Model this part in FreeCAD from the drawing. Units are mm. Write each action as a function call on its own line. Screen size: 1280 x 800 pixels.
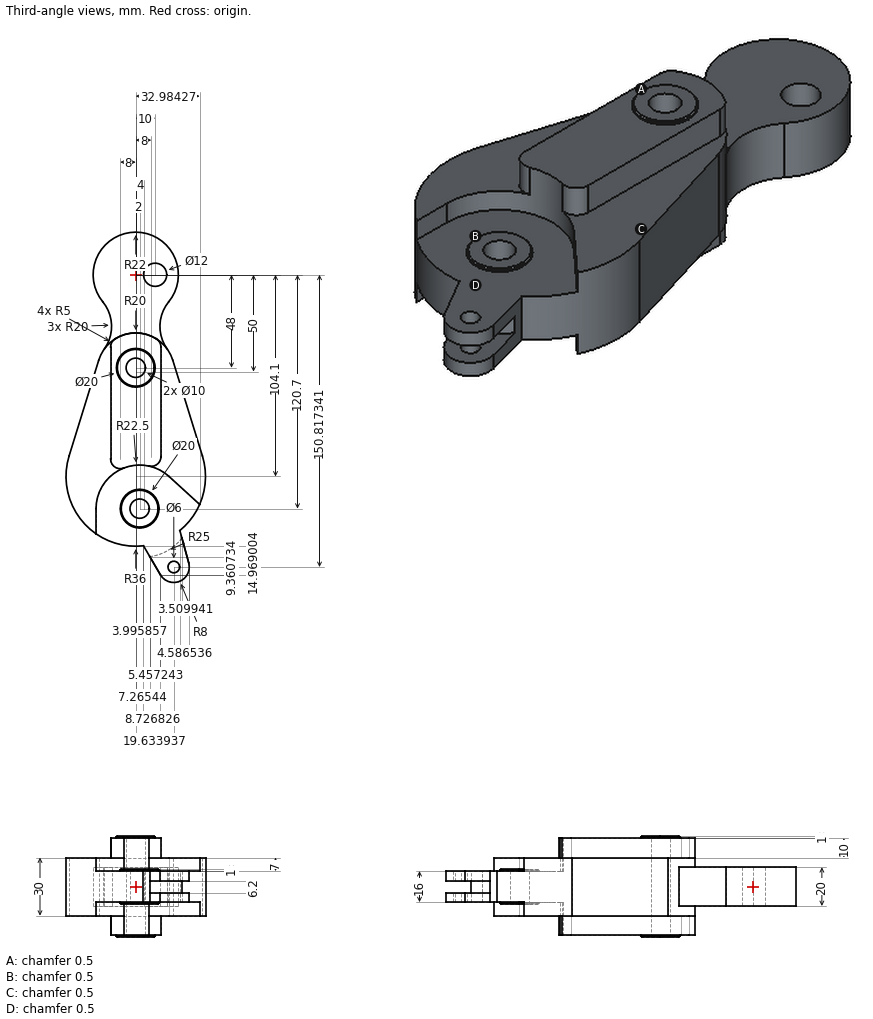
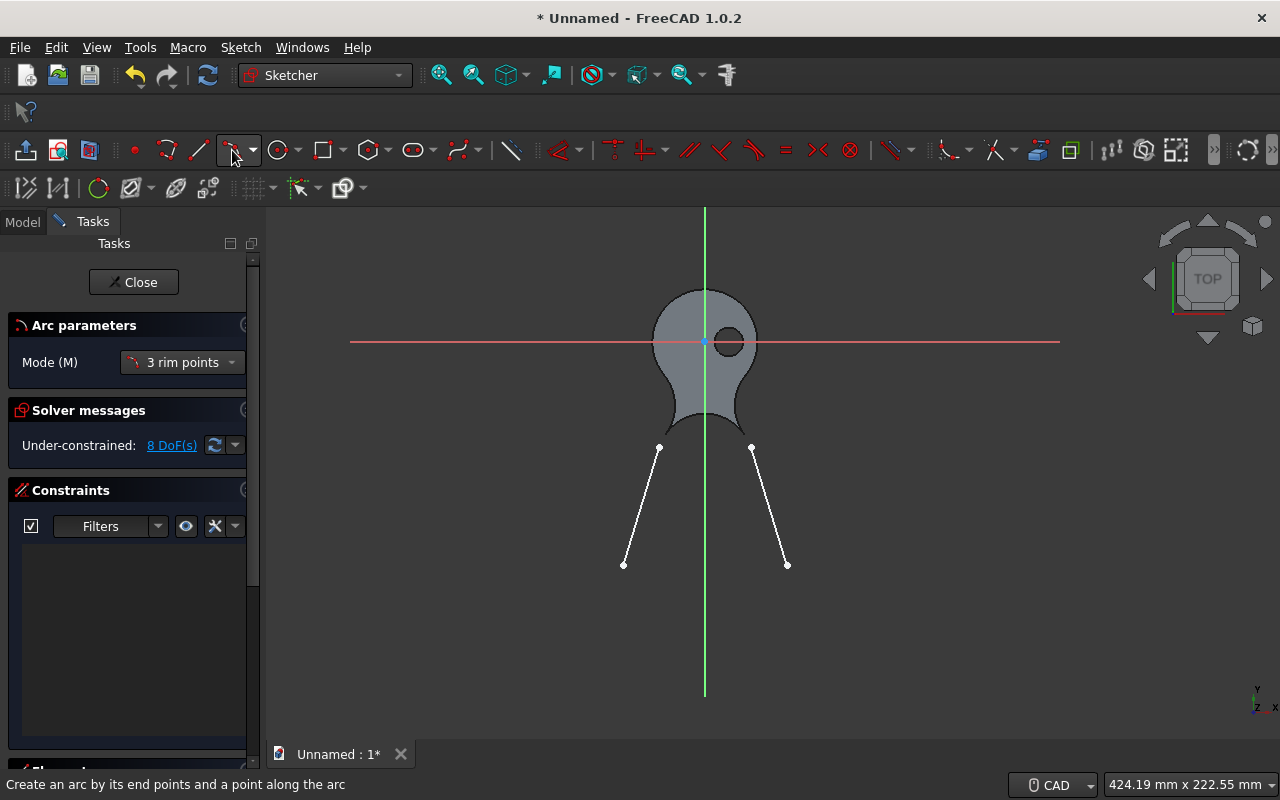
click(623, 566)
click(787, 566)
click(673, 671)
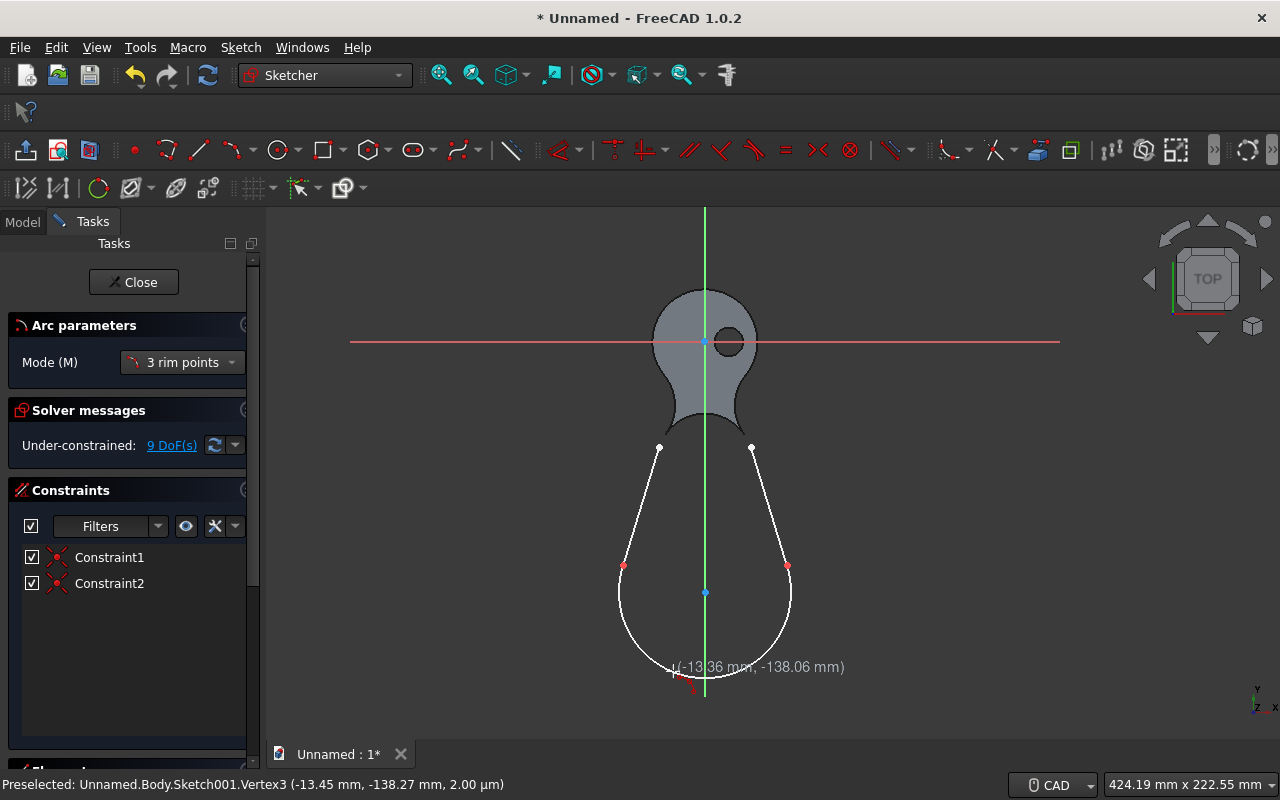
click(751, 448)
click(659, 448)
click(728, 420)
key(Escape)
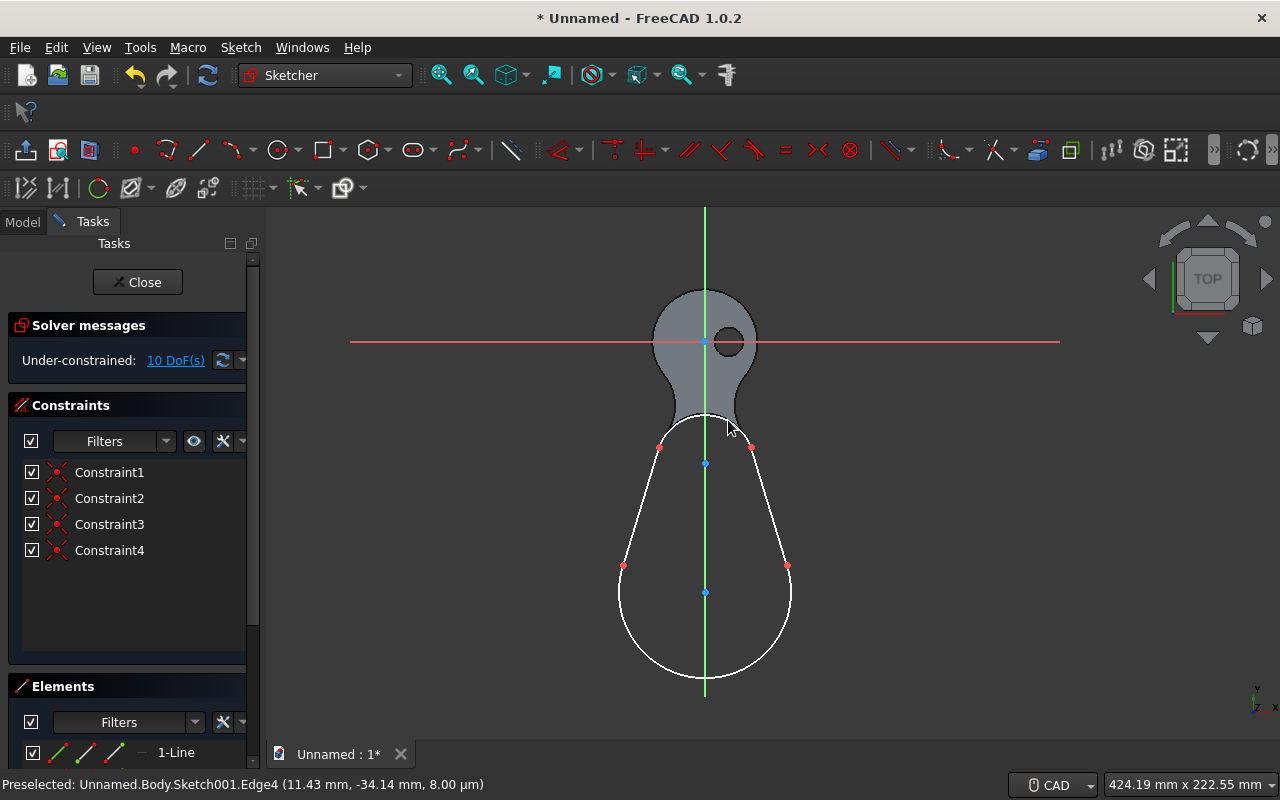
click(648, 483)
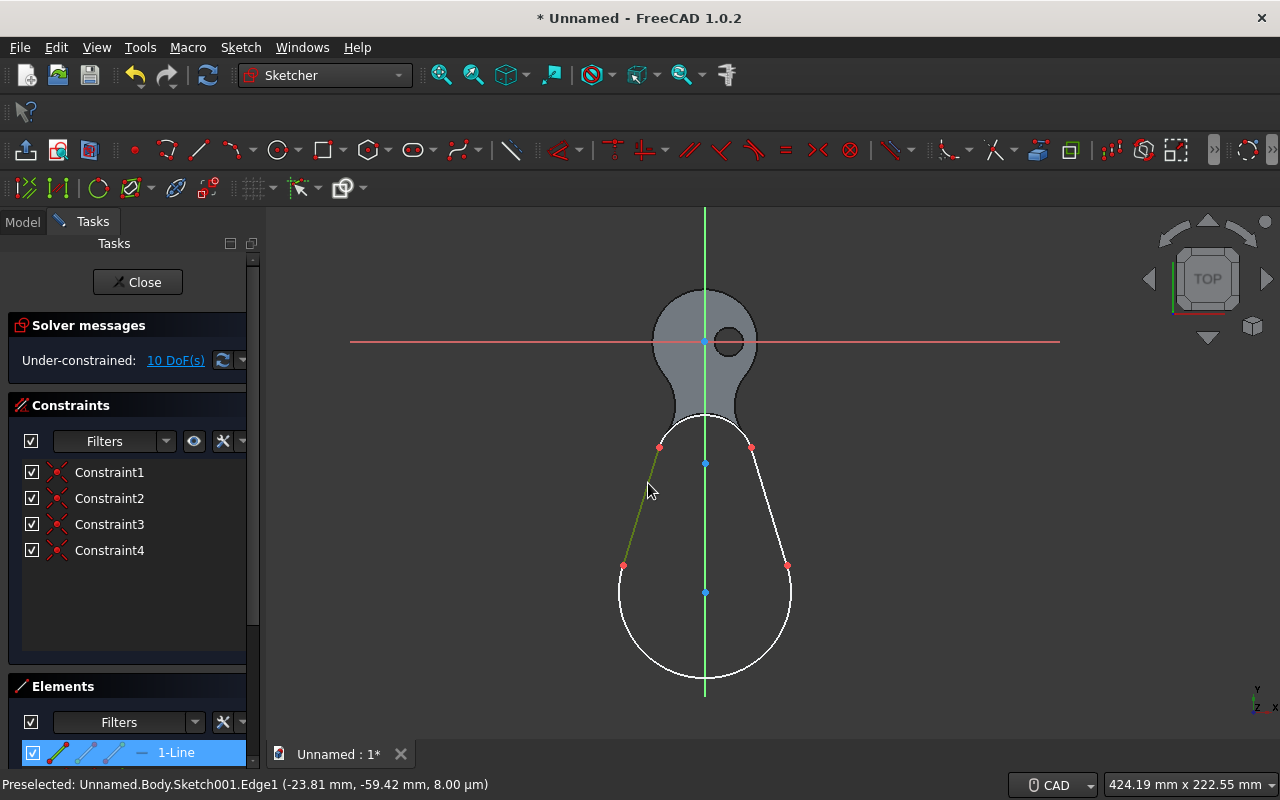
click(646, 655)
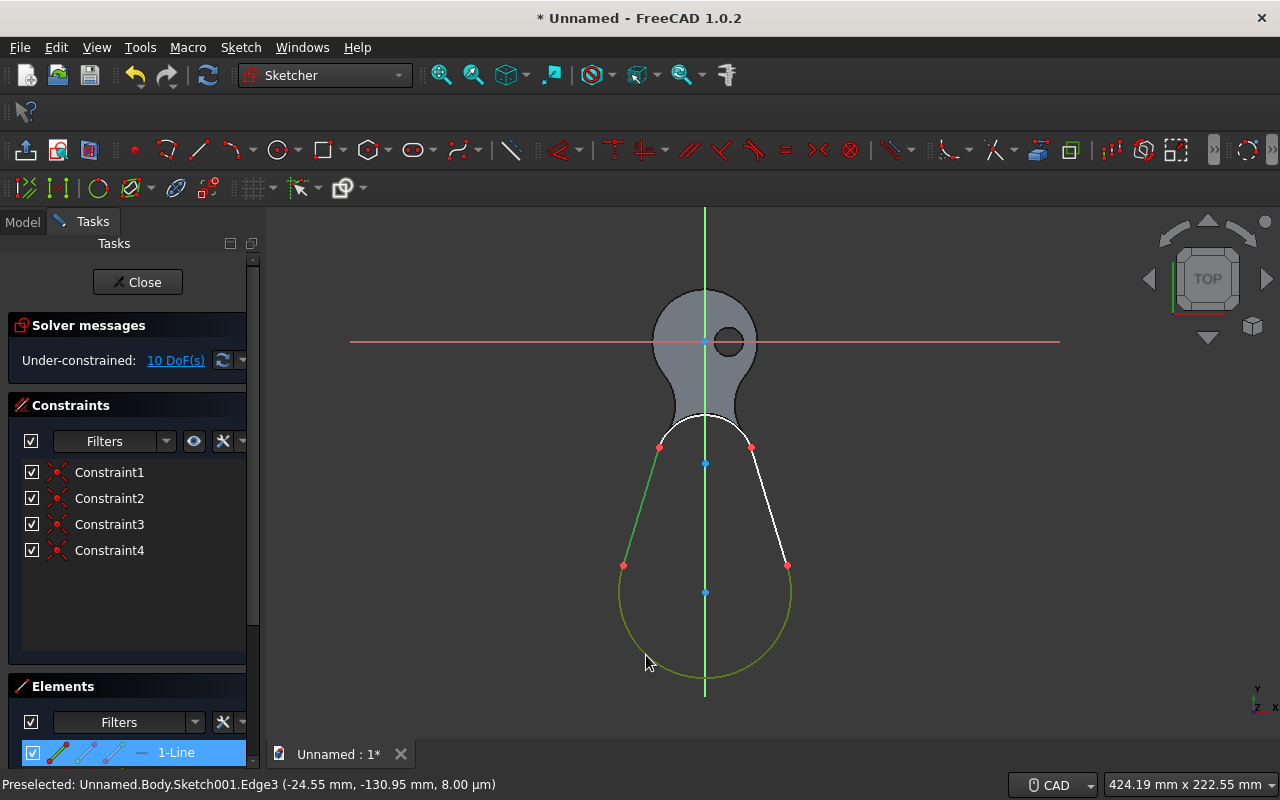
click(754, 150)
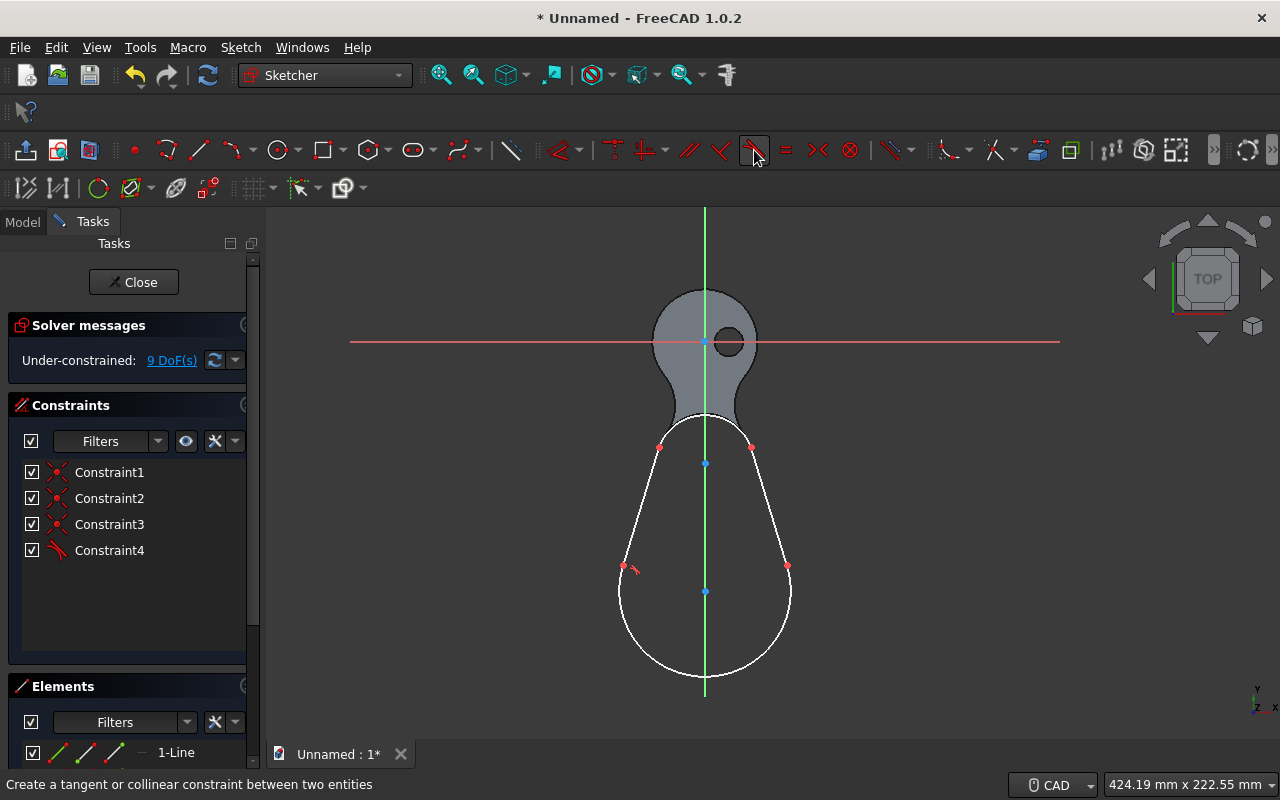
click(648, 483)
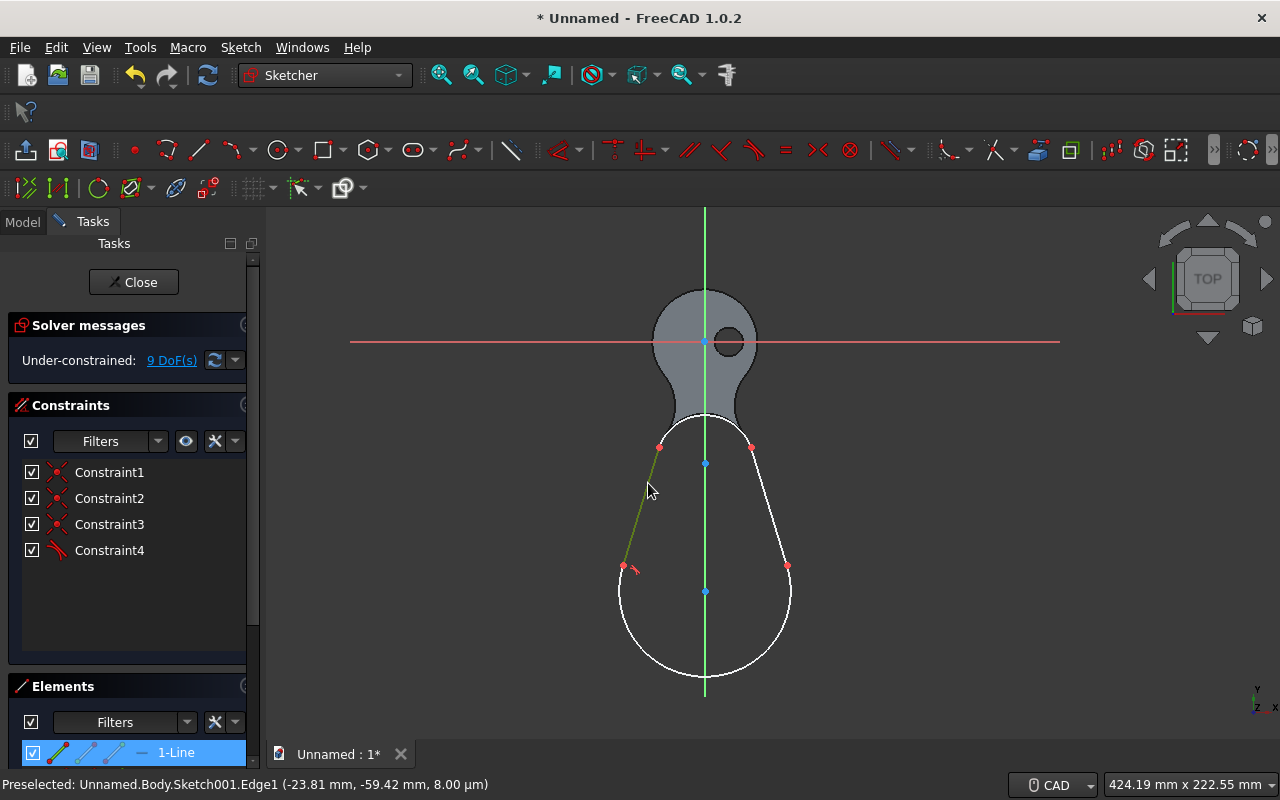
click(728, 421)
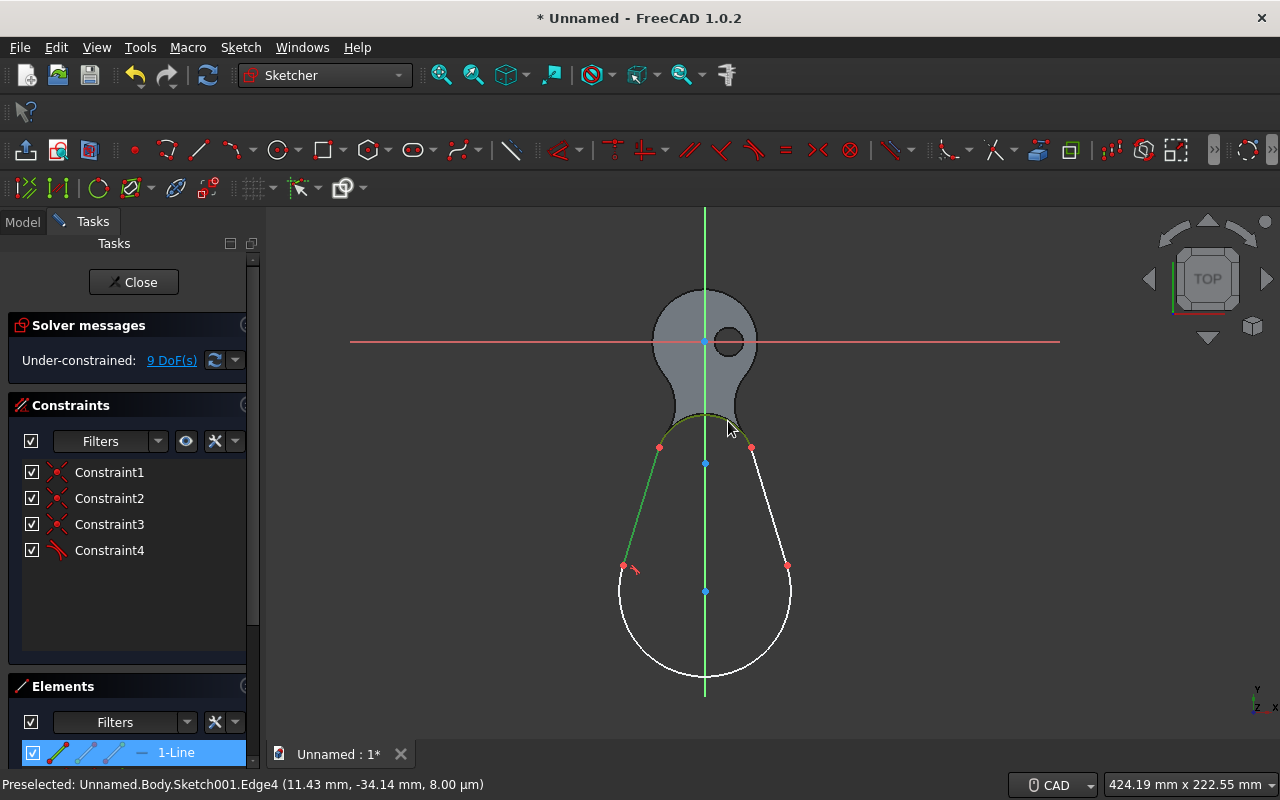
click(754, 150)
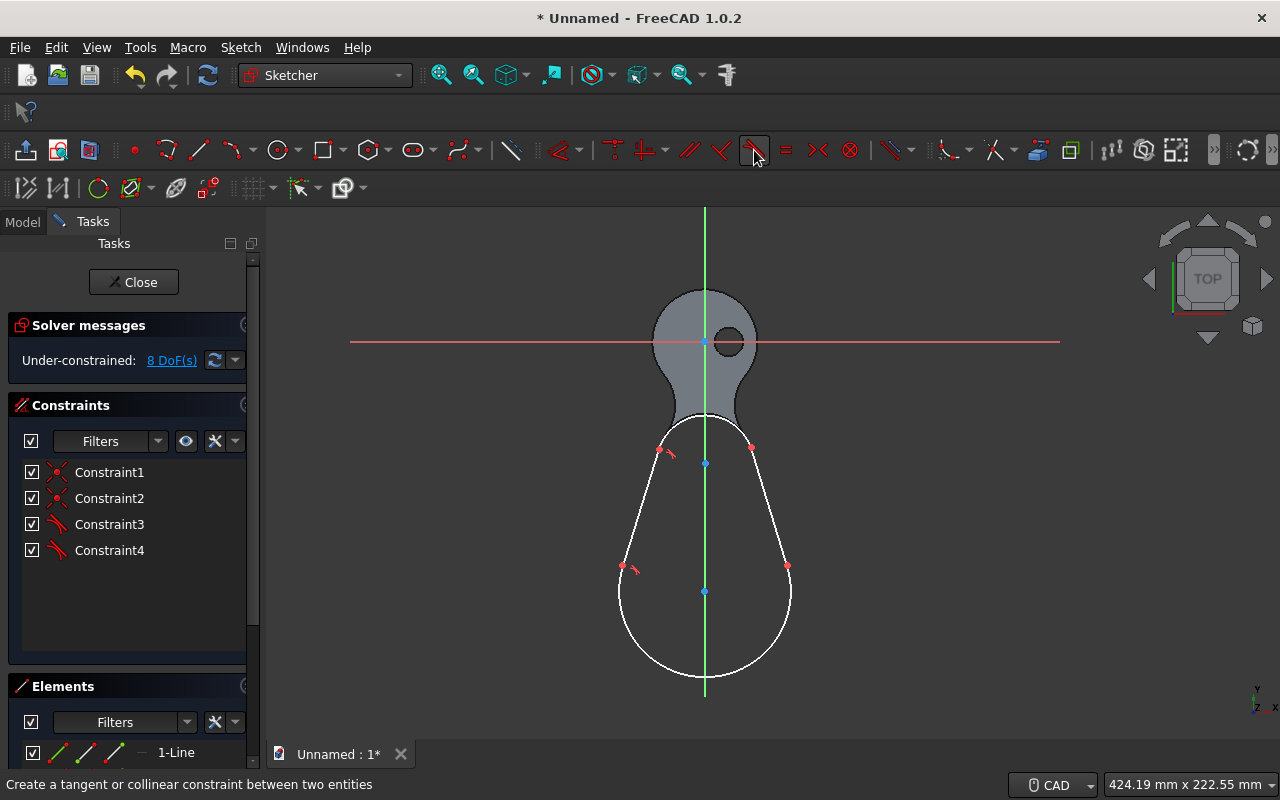
click(776, 531)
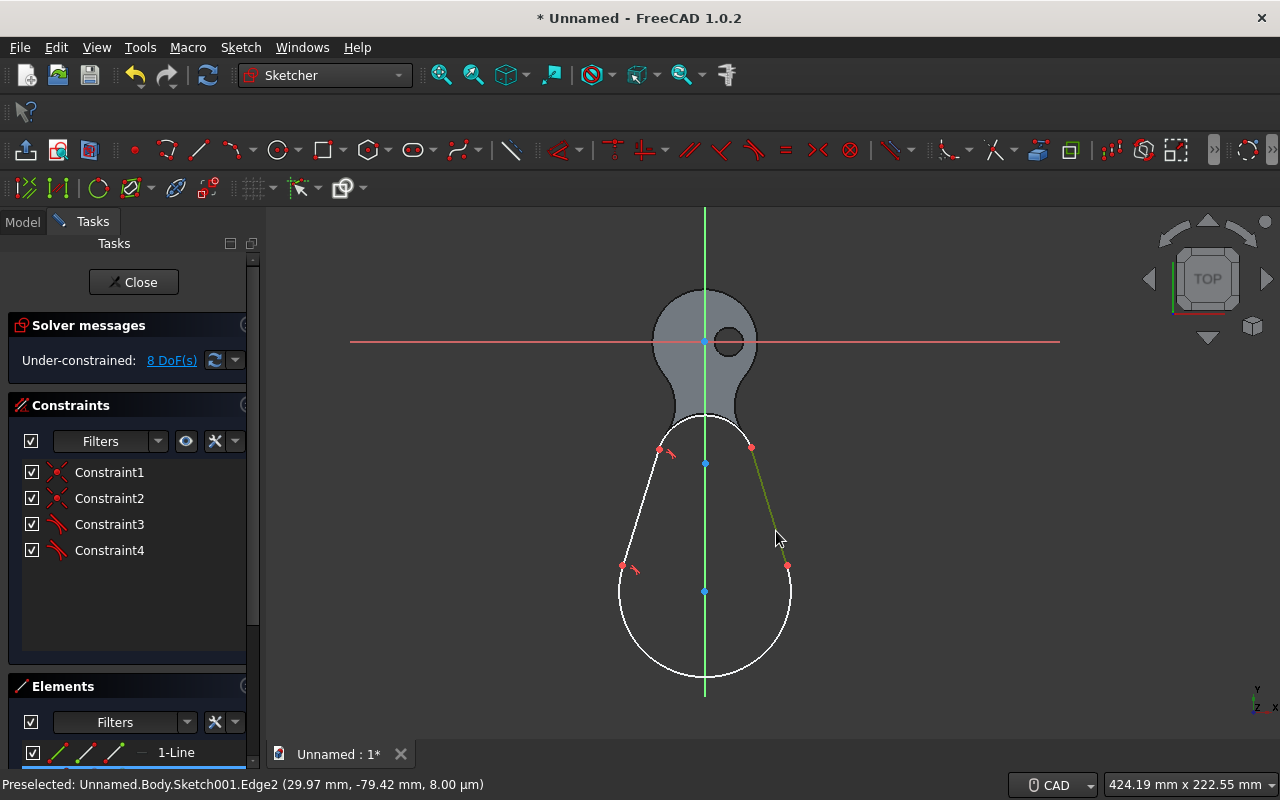
click(647, 654)